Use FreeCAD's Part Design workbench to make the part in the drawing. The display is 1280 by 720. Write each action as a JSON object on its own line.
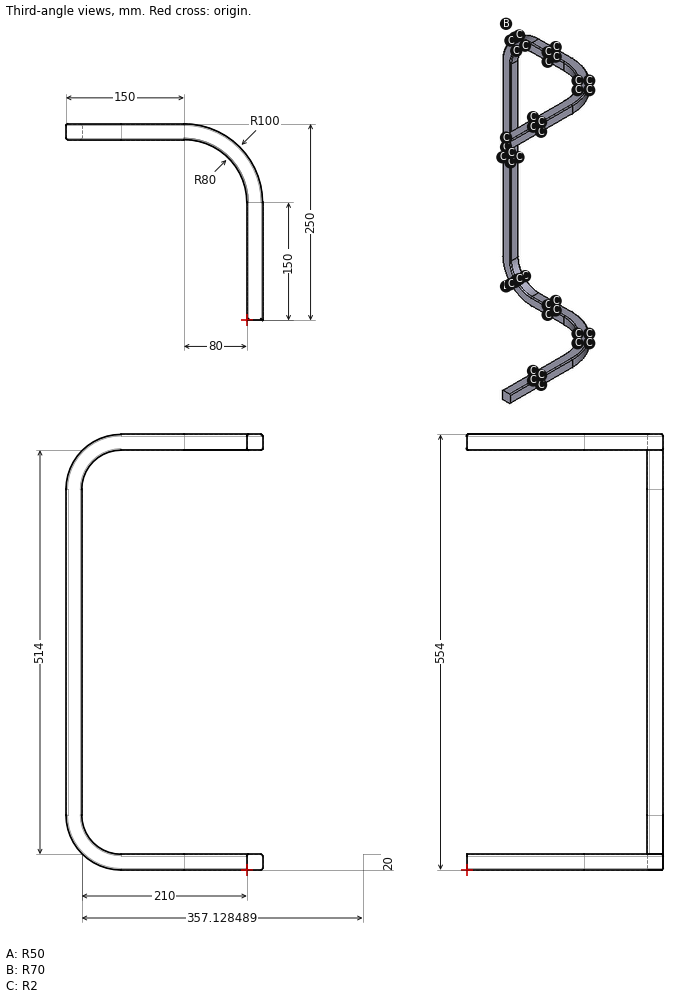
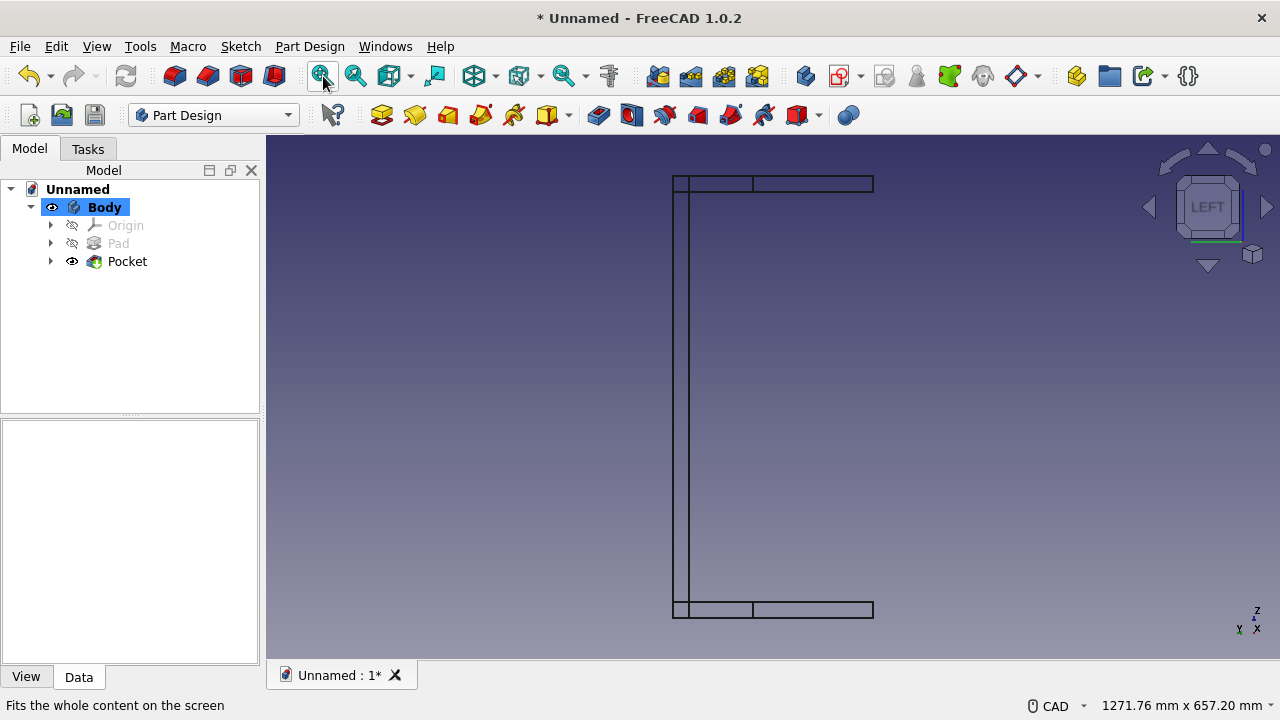
{"action": "key", "text": "0"}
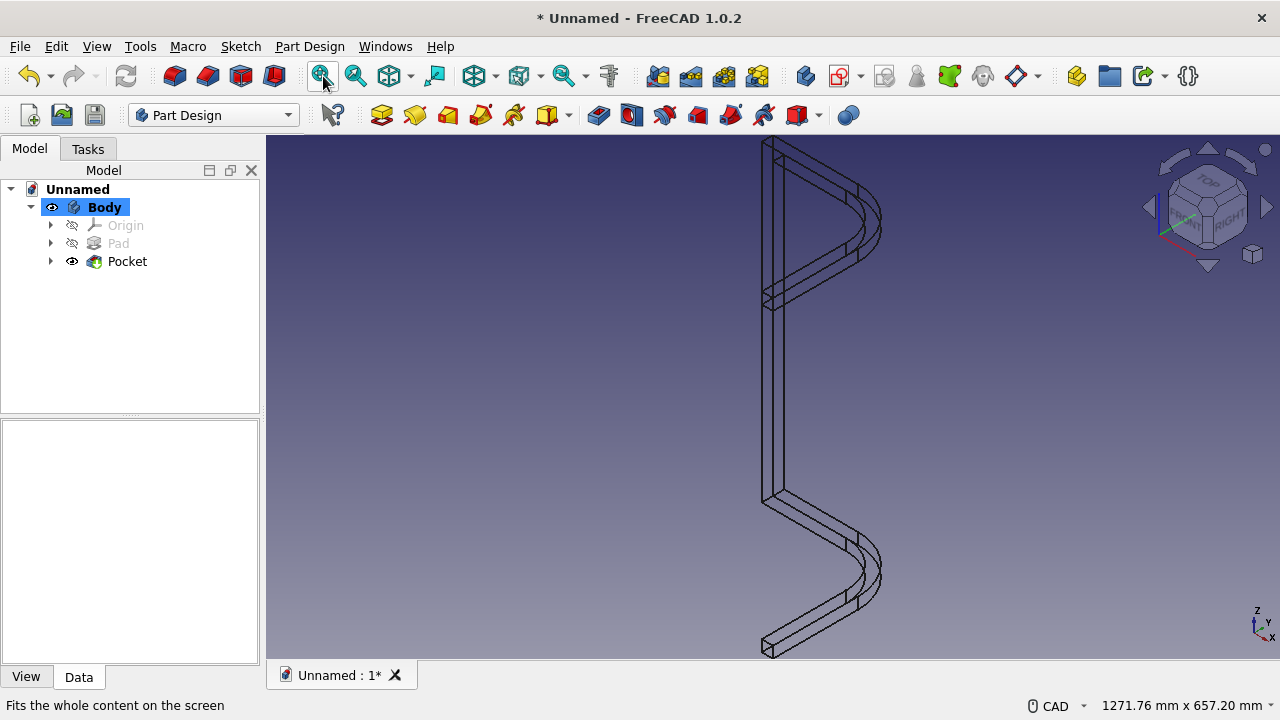
{"action": "left_click", "coordinate": [323, 76]}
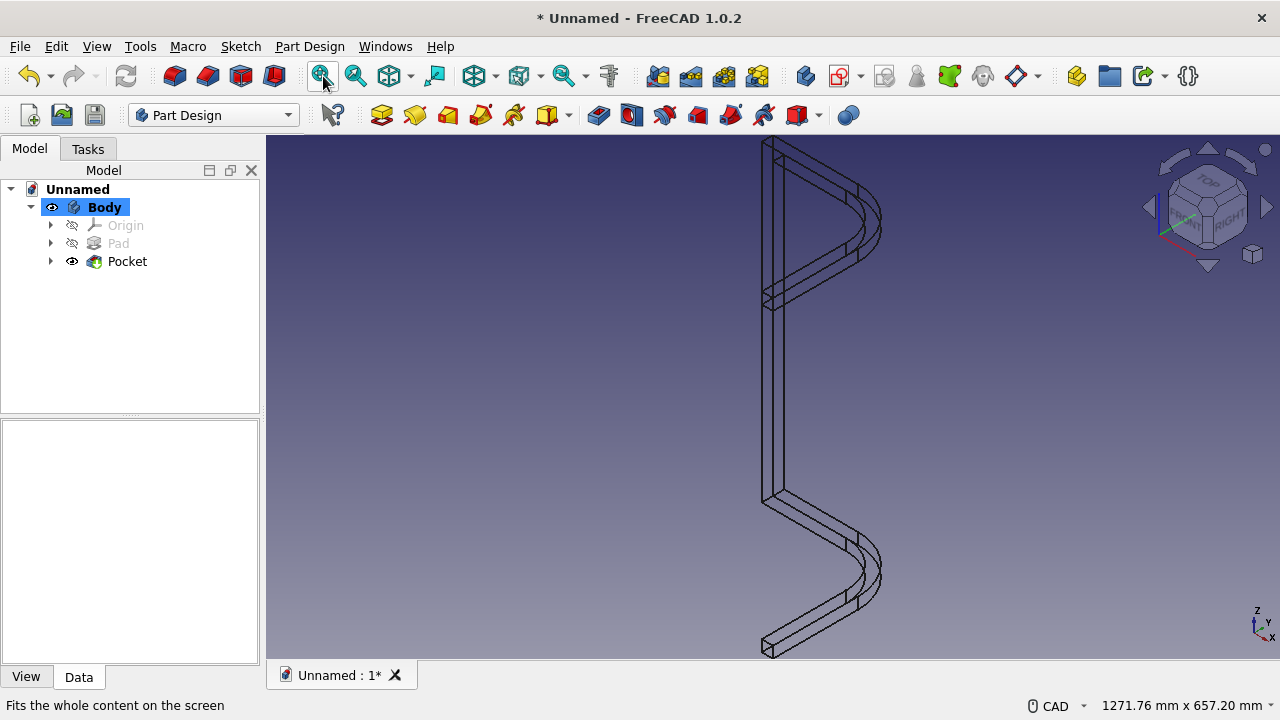
{"action": "left_click", "coordinate": [780, 491]}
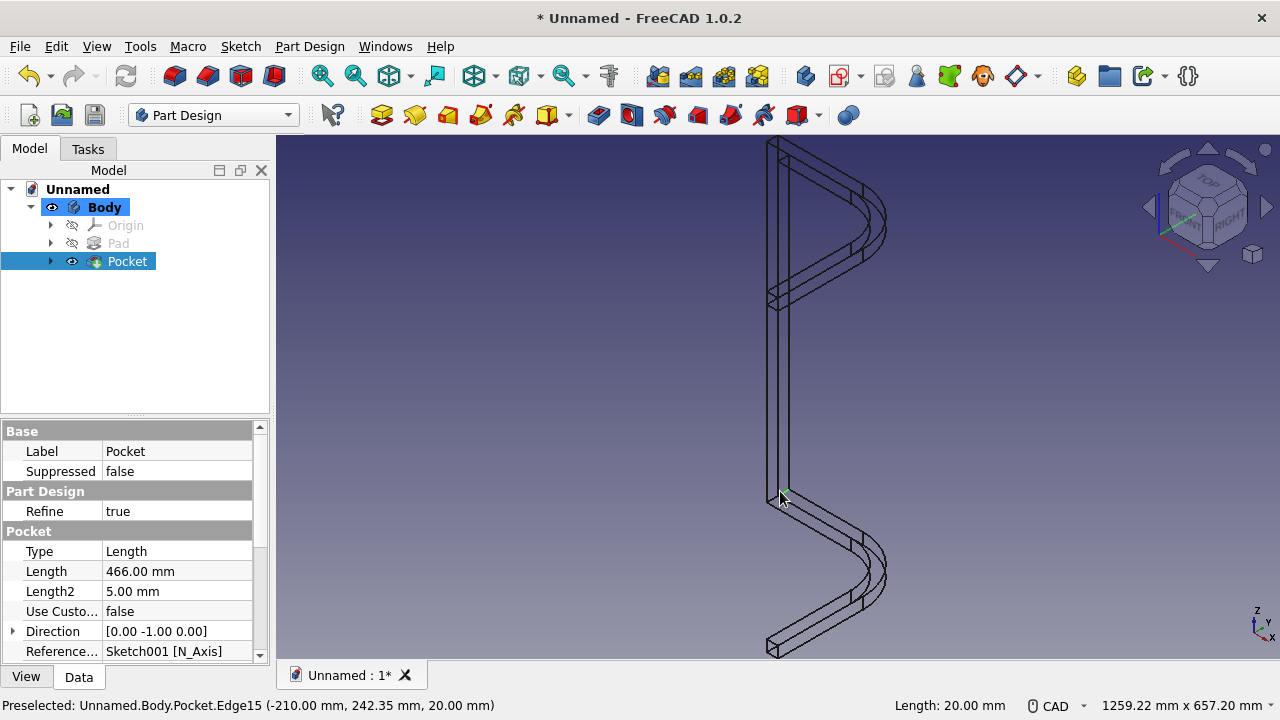
{"action": "key", "text": "2"}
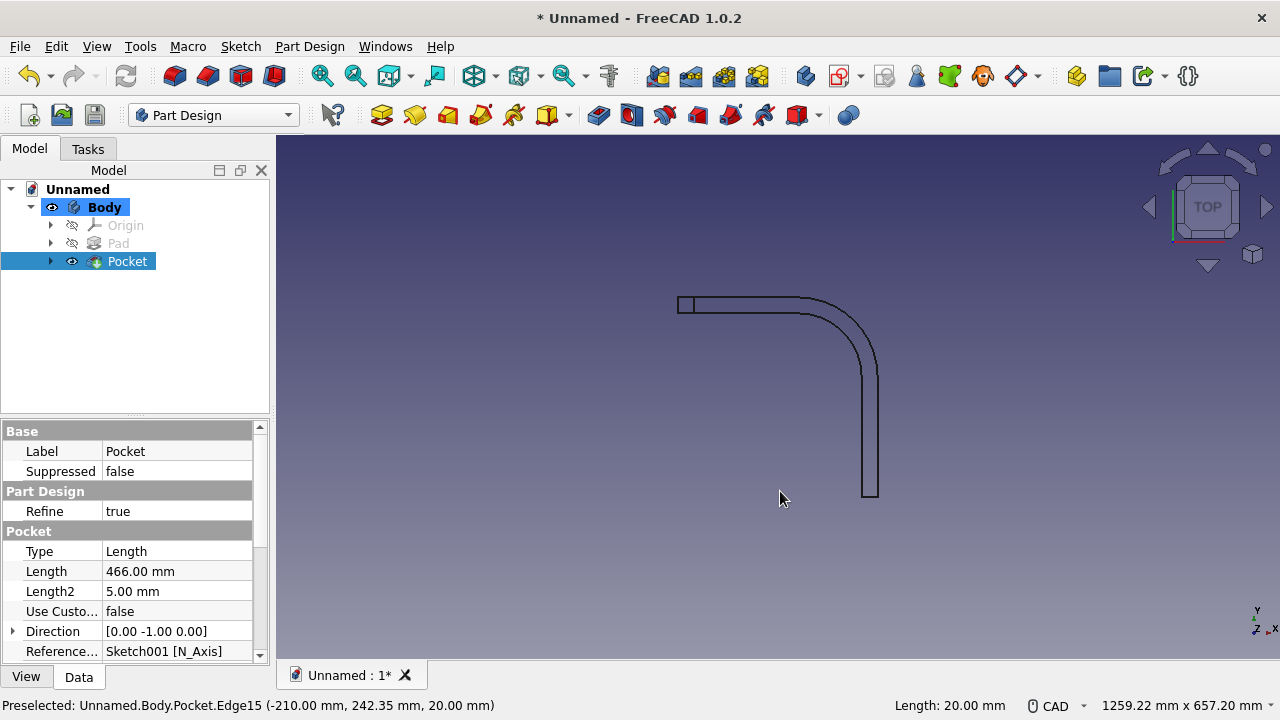
{"action": "left_click", "coordinate": [323, 76]}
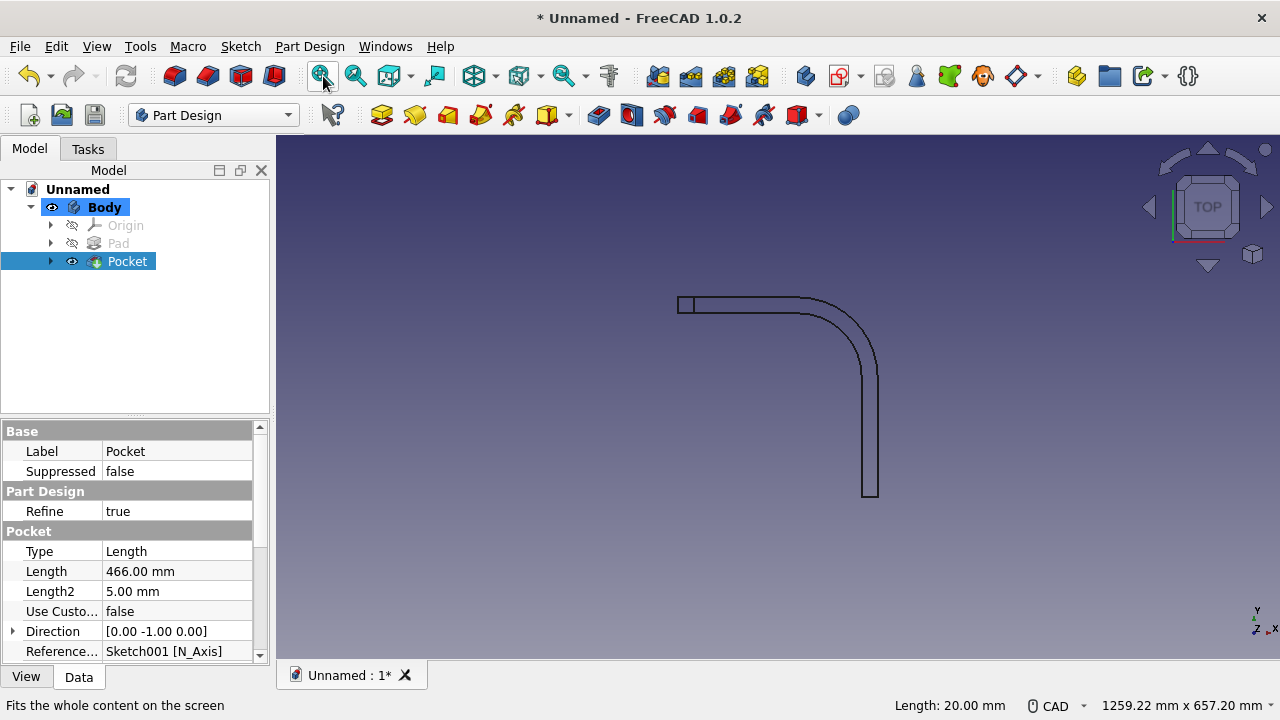
{"action": "left_click", "coordinate": [694, 304], "text": "ctrl"}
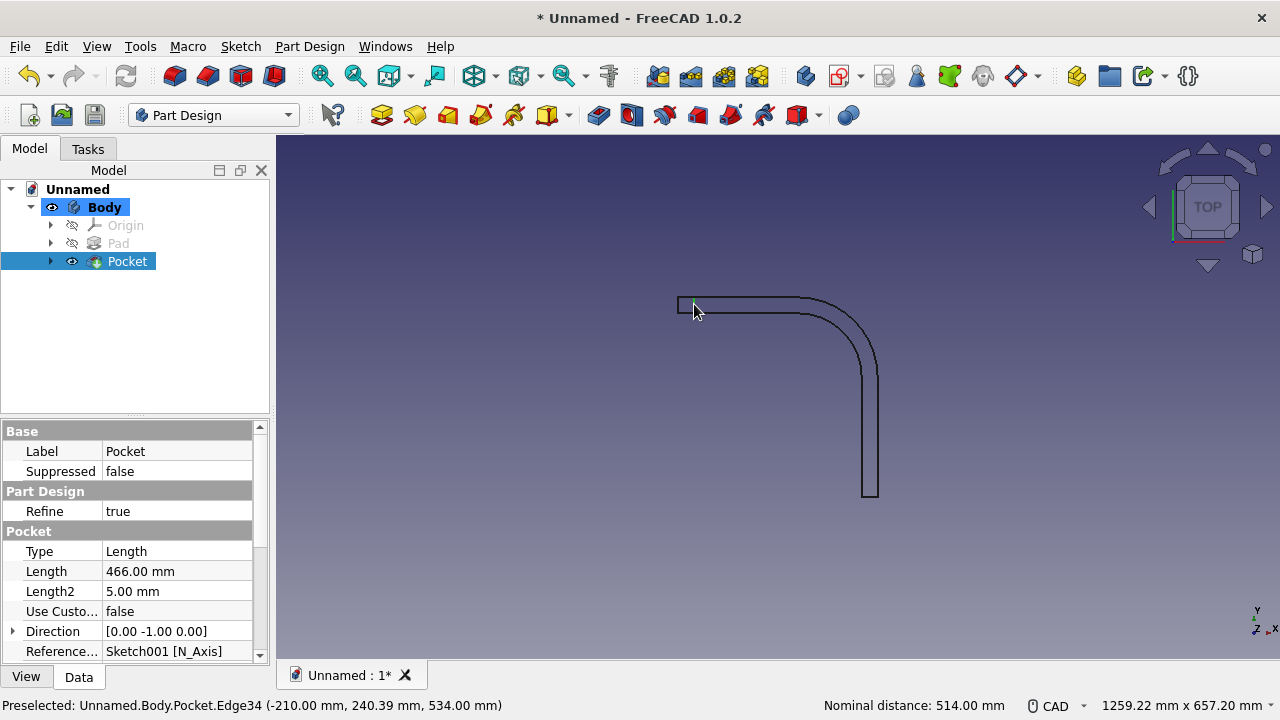
{"action": "key", "text": "v 1"}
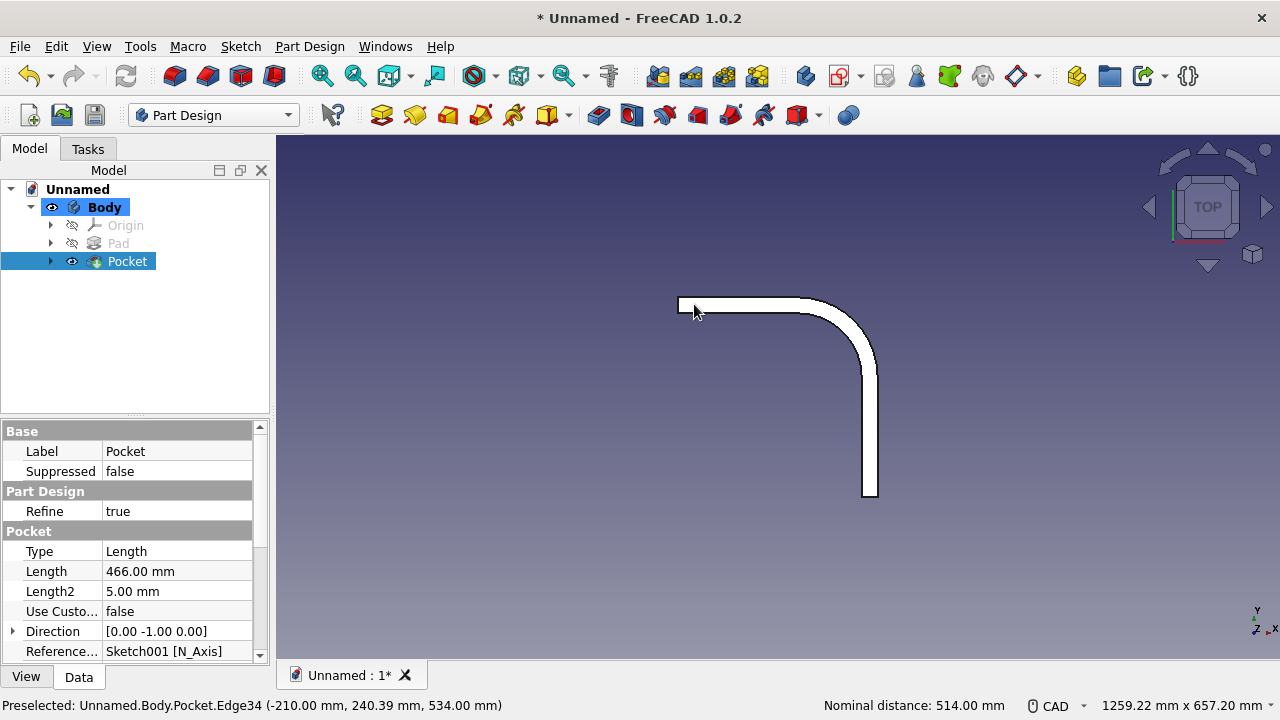
{"action": "left_click", "coordinate": [175, 76]}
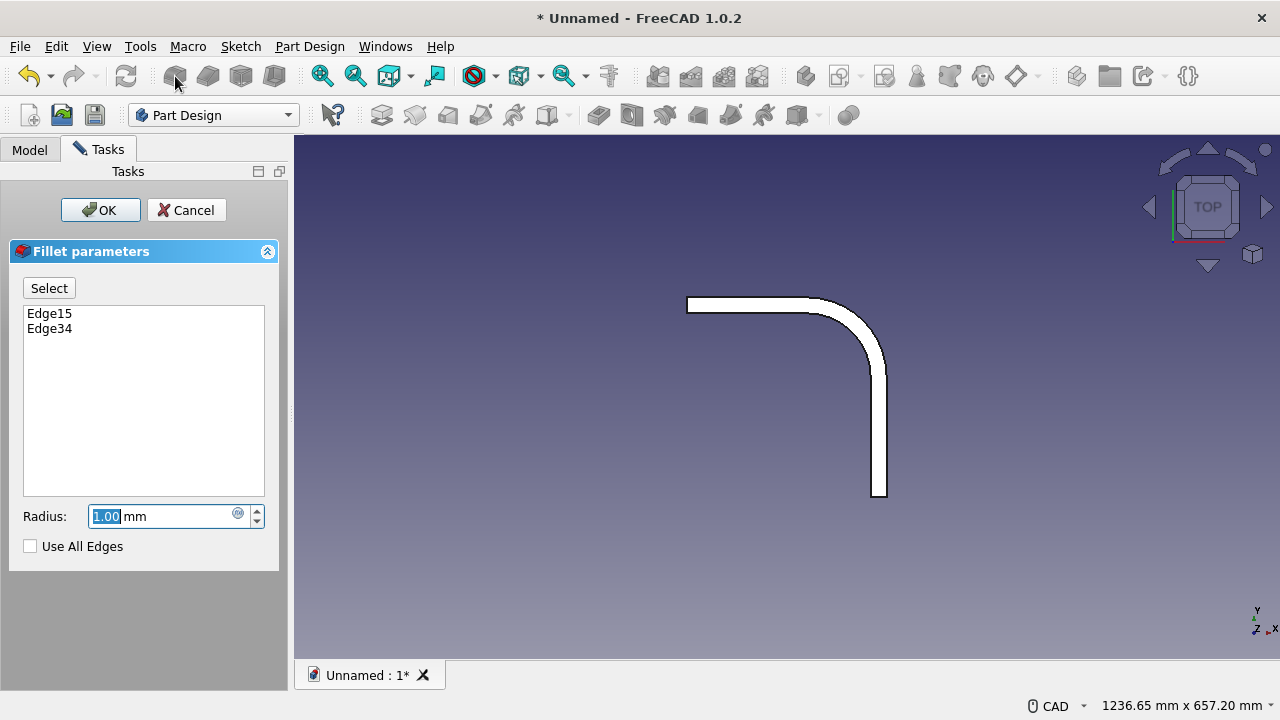
{"action": "type", "text": "50"}
{"action": "key", "text": "Tab"}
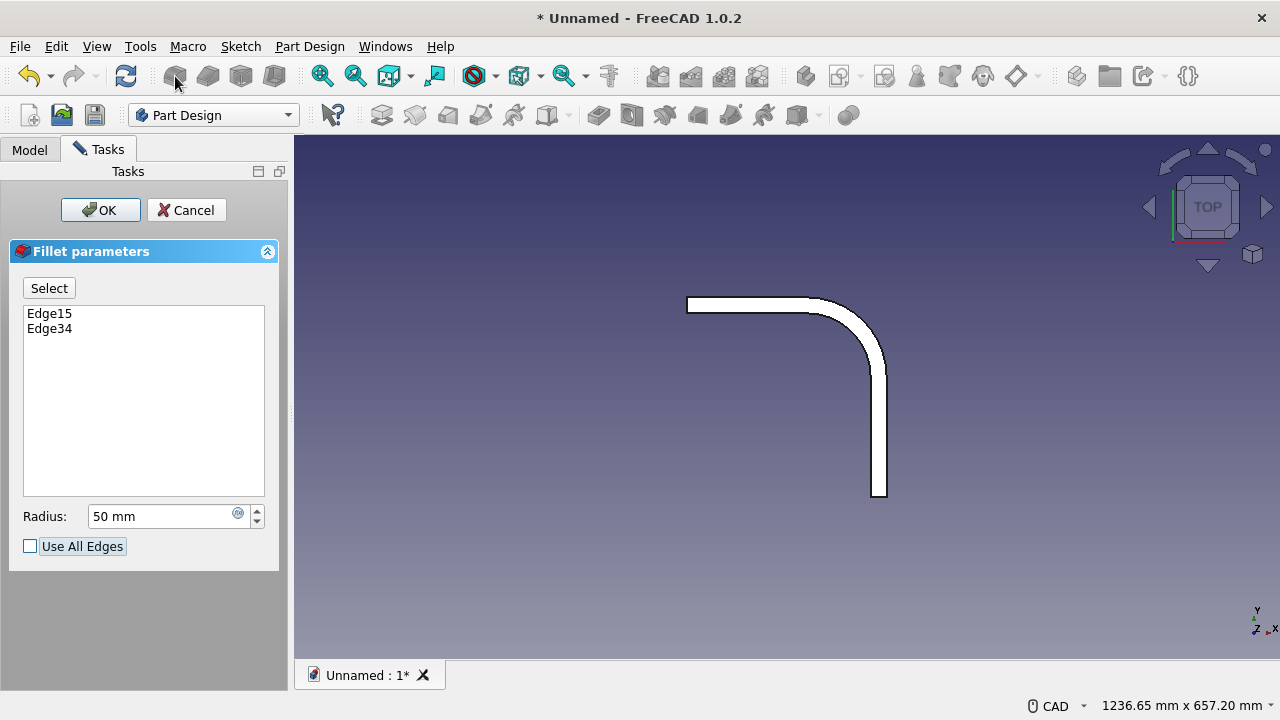
{"action": "left_click", "coordinate": [101, 210]}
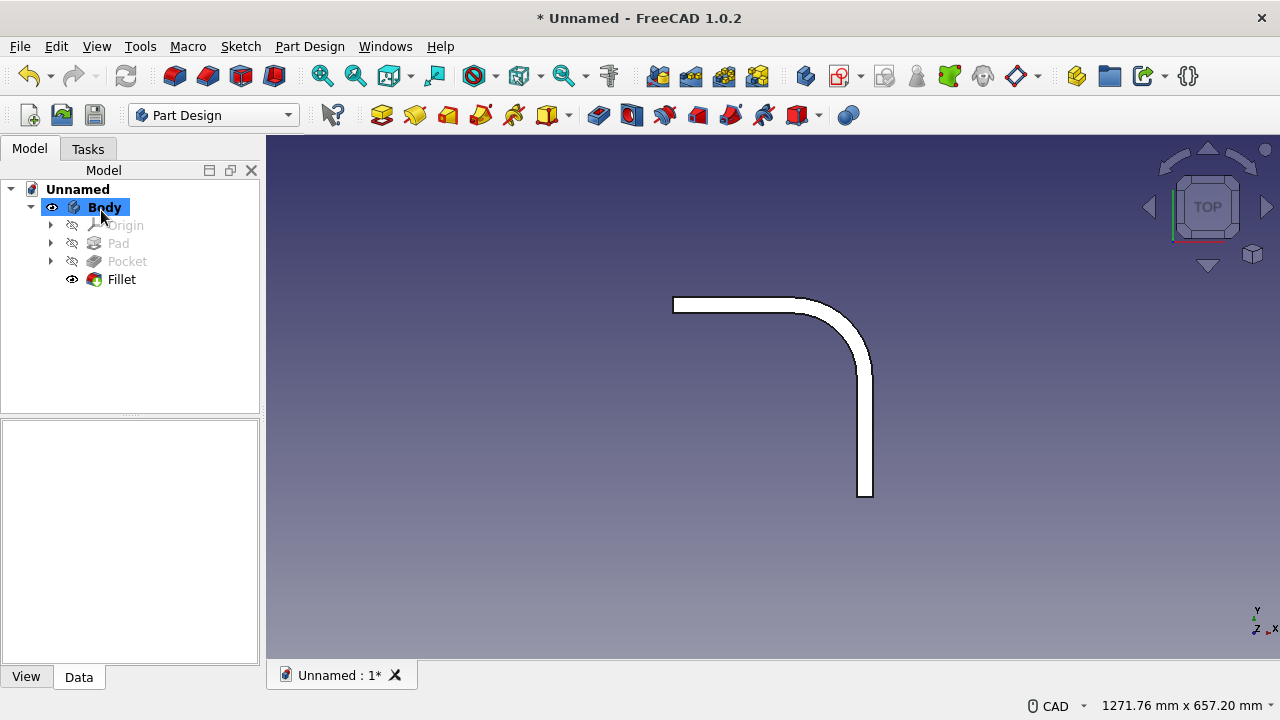
{"action": "left_click", "coordinate": [323, 76]}